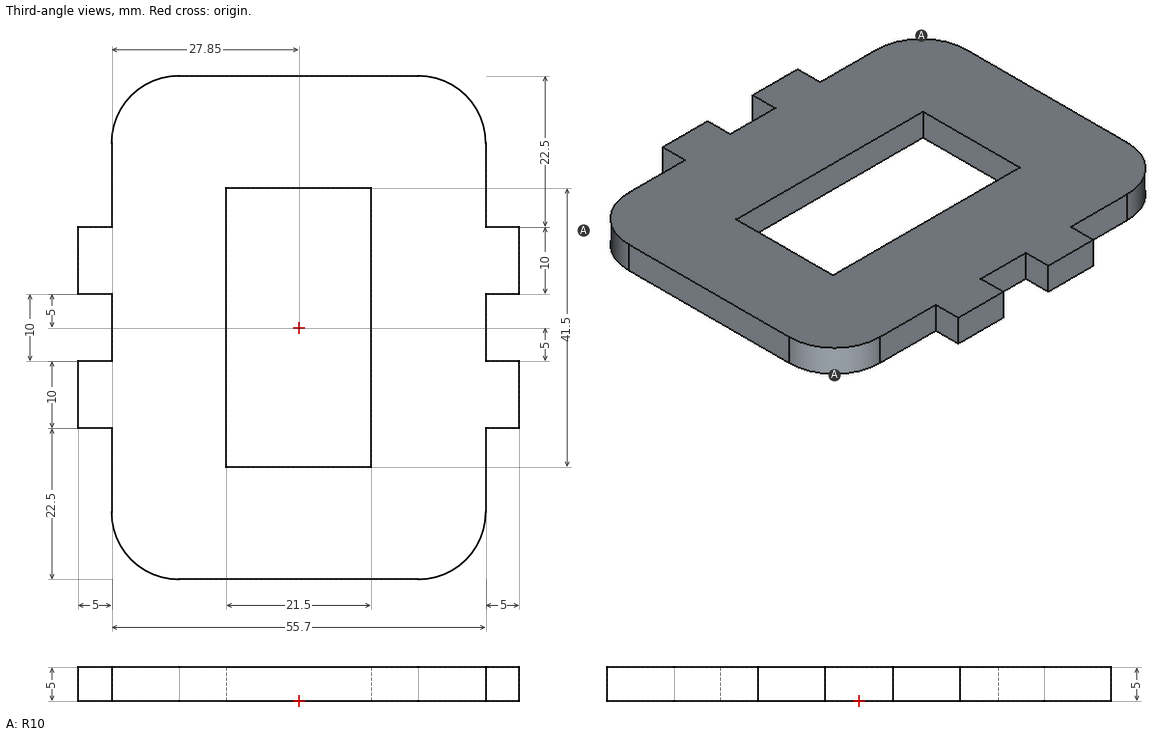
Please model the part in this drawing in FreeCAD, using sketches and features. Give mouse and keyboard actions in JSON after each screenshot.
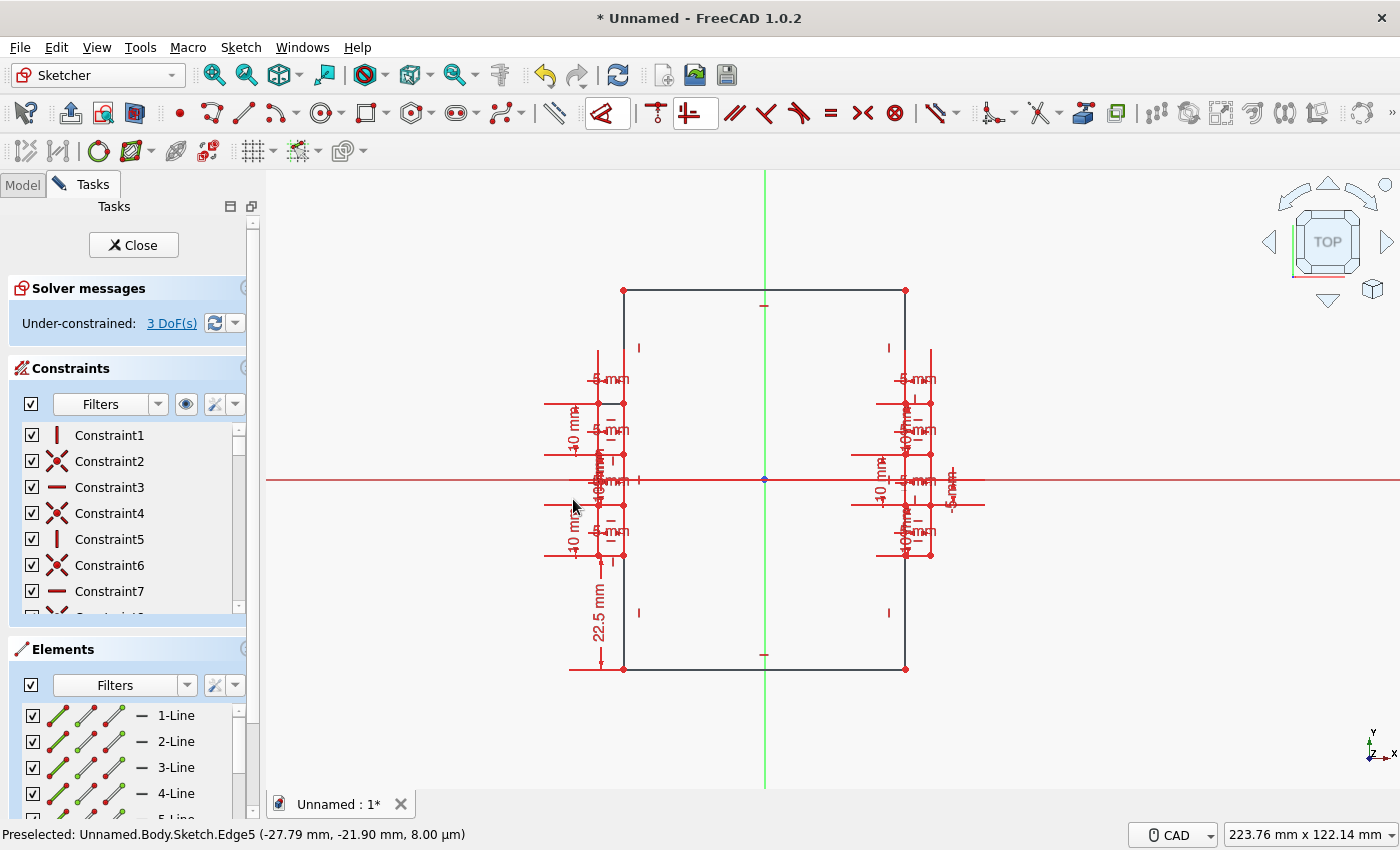
{"action": "left_click", "coordinate": [708, 670]}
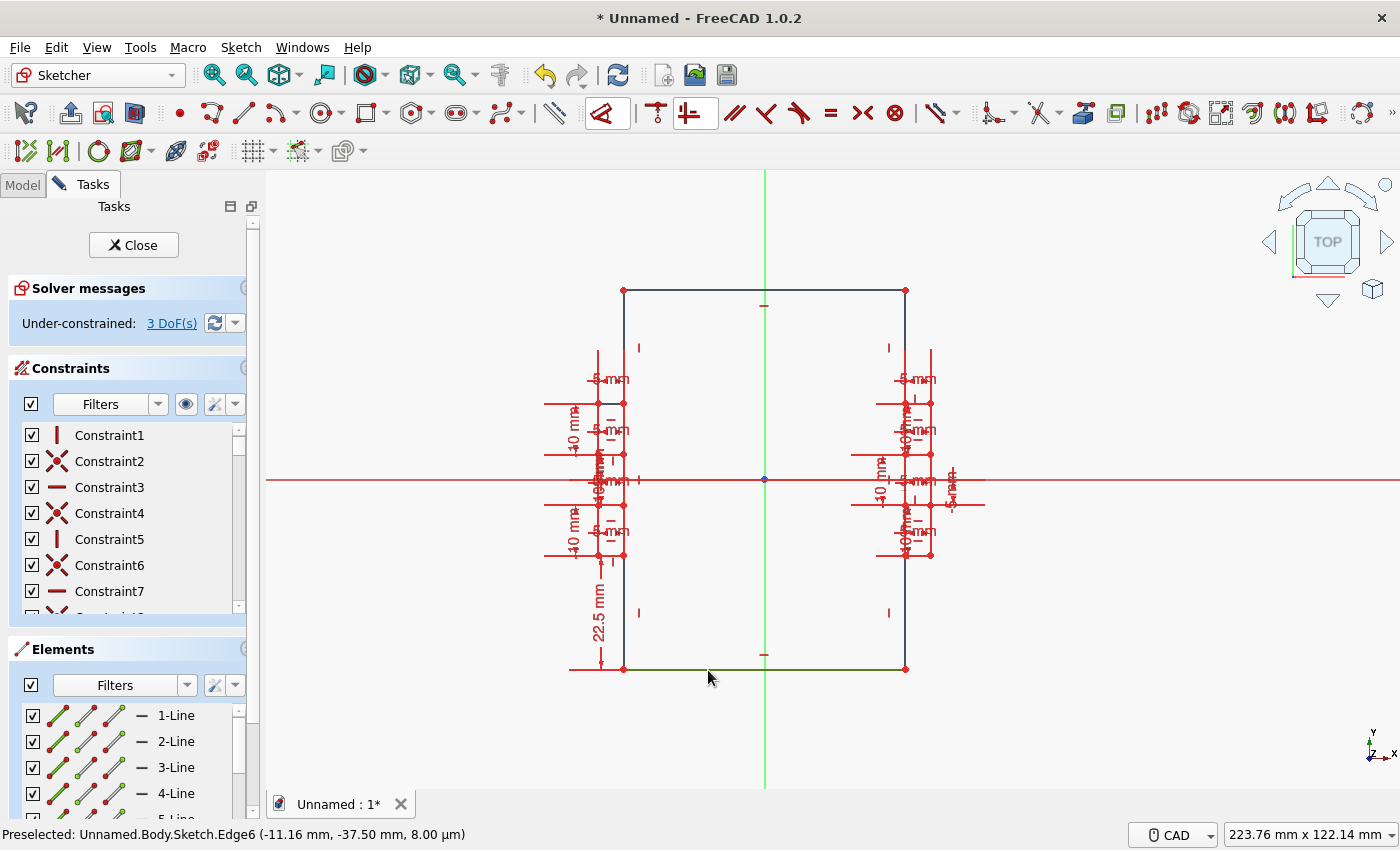
{"action": "left_click", "coordinate": [624, 114]}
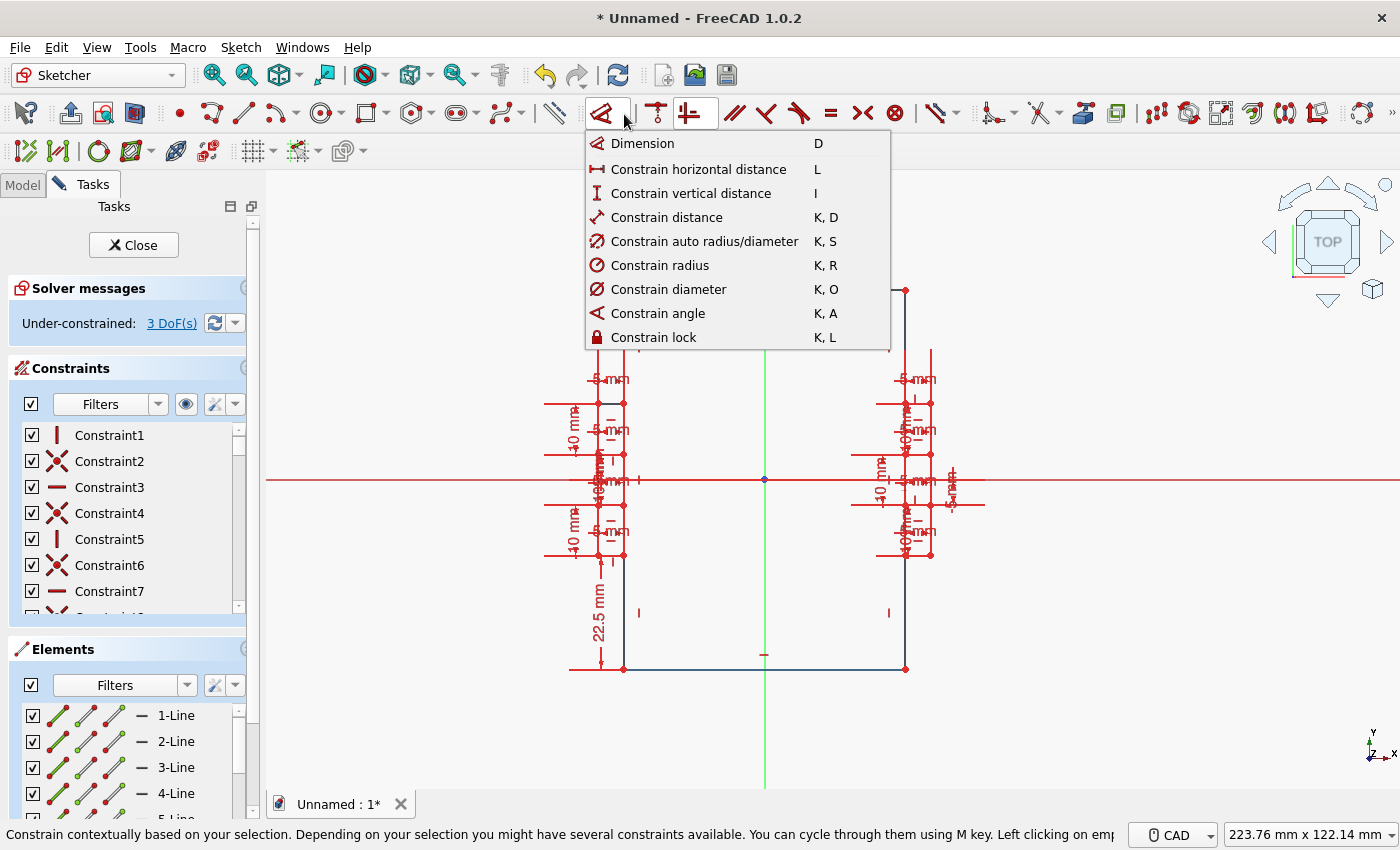
{"action": "left_click", "coordinate": [738, 169]}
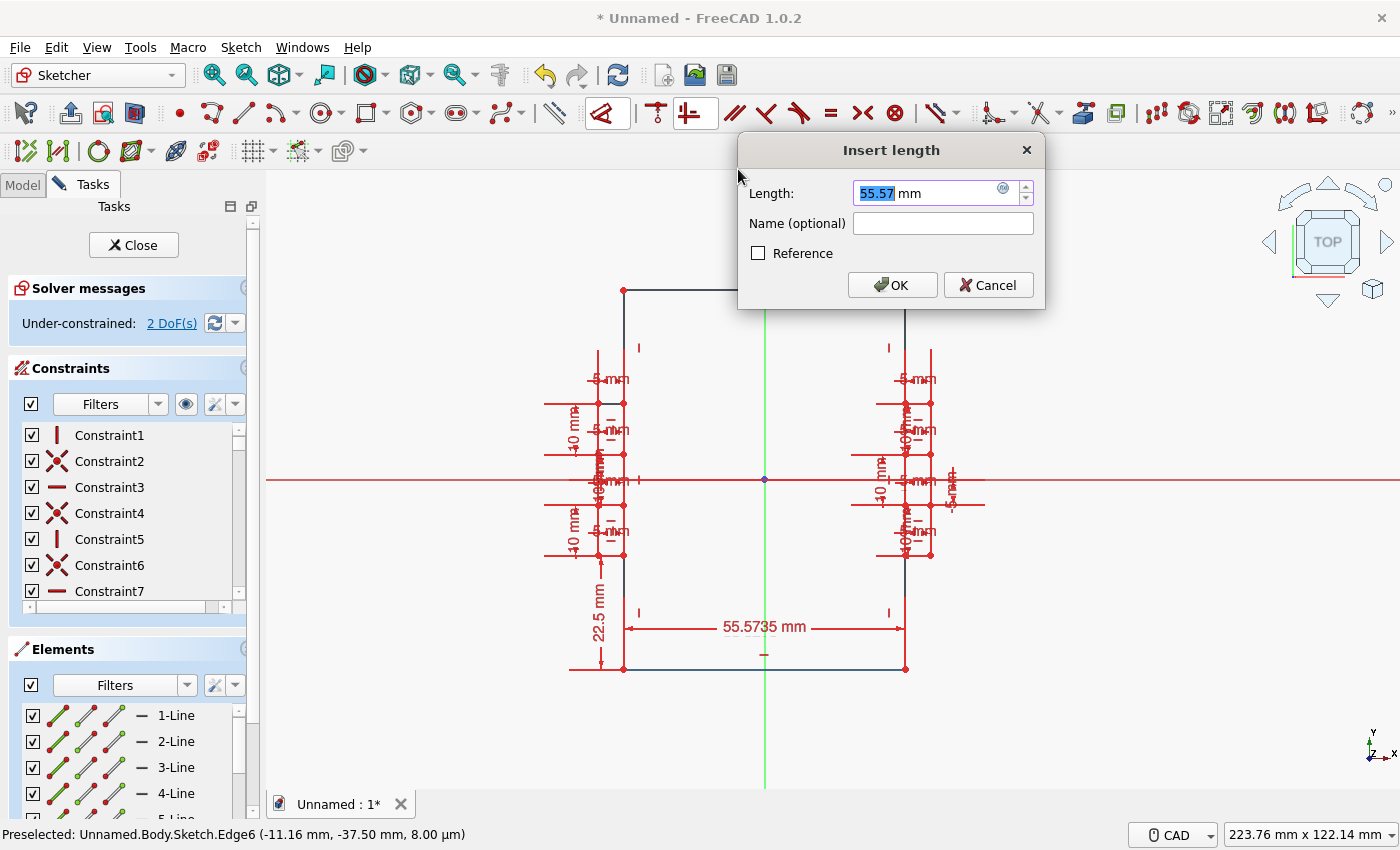
{"action": "type", "text": "55.7"}
{"action": "key", "text": "Return"}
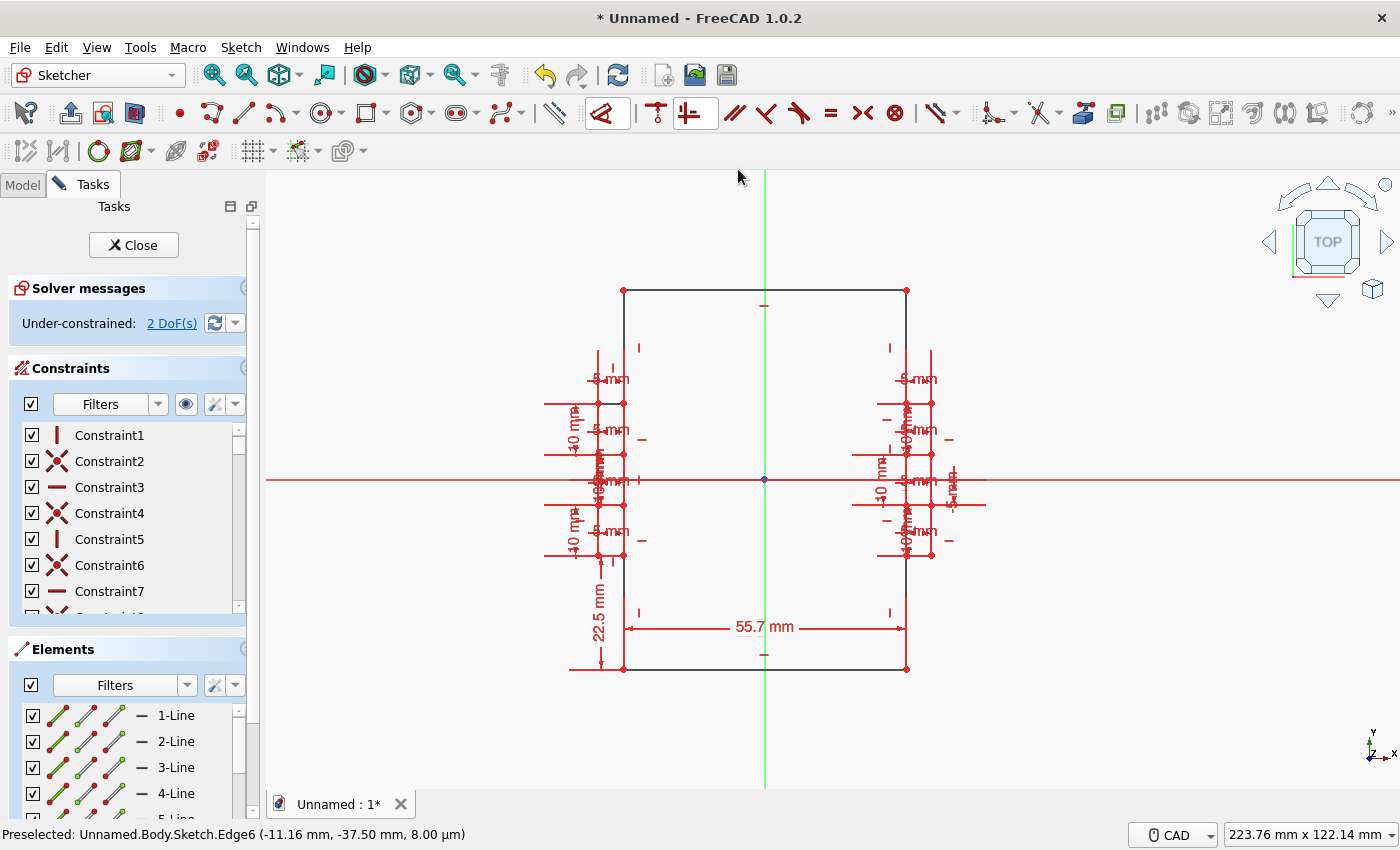
{"action": "left_click", "coordinate": [906, 370]}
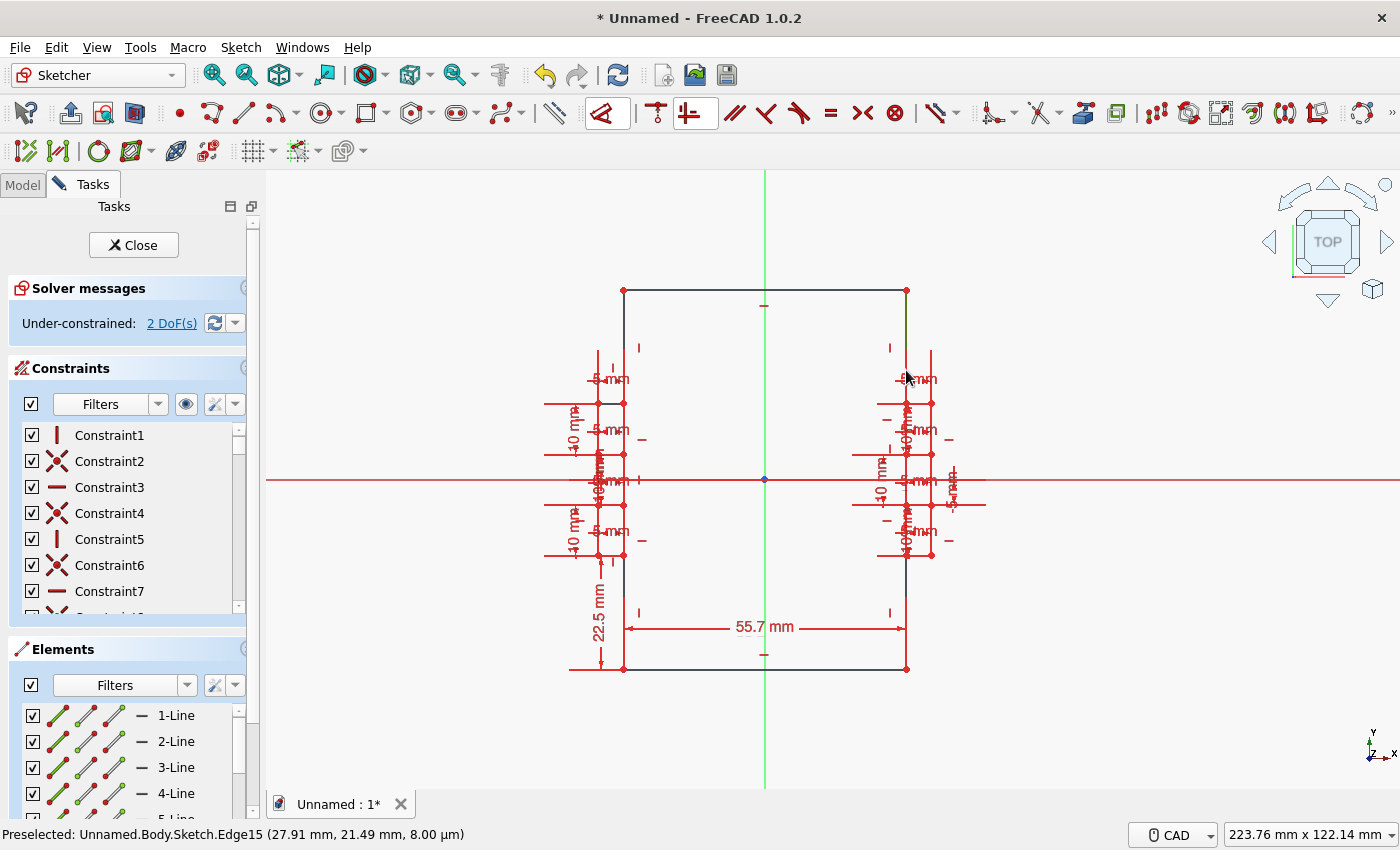
{"action": "left_click", "coordinate": [624, 114]}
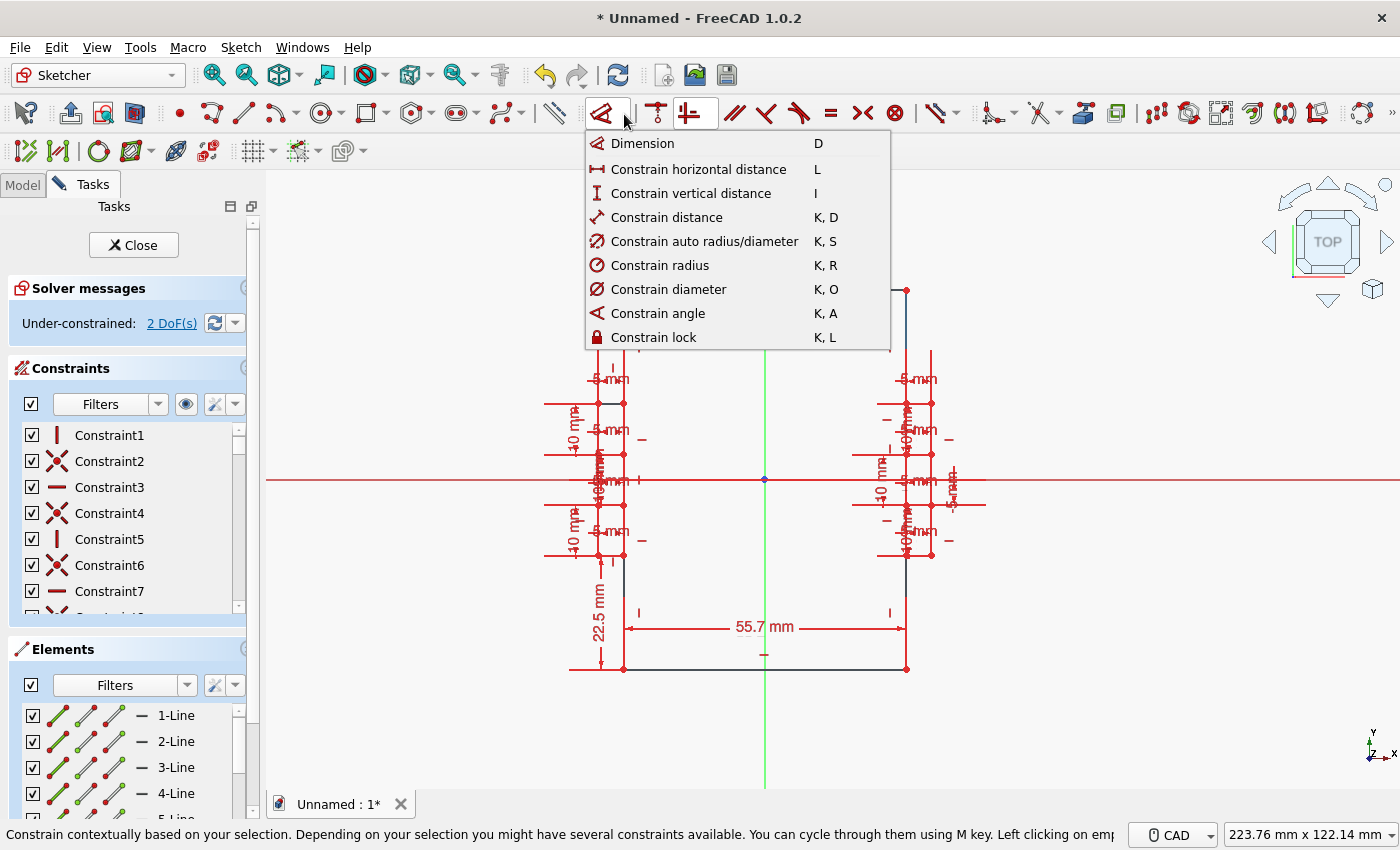
{"action": "left_click", "coordinate": [738, 193]}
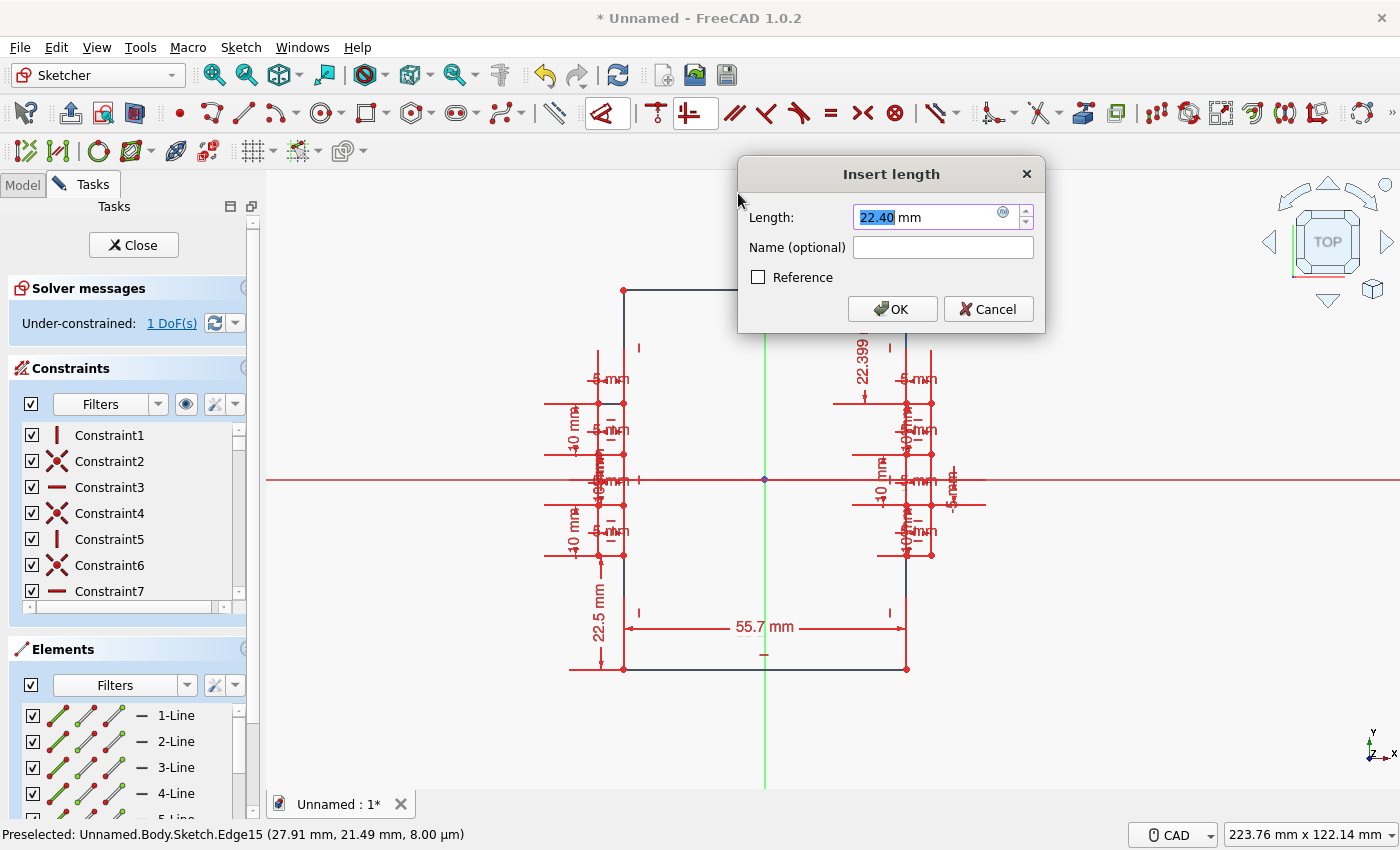
{"action": "type", "text": "22.5"}
{"action": "key", "text": "Return"}